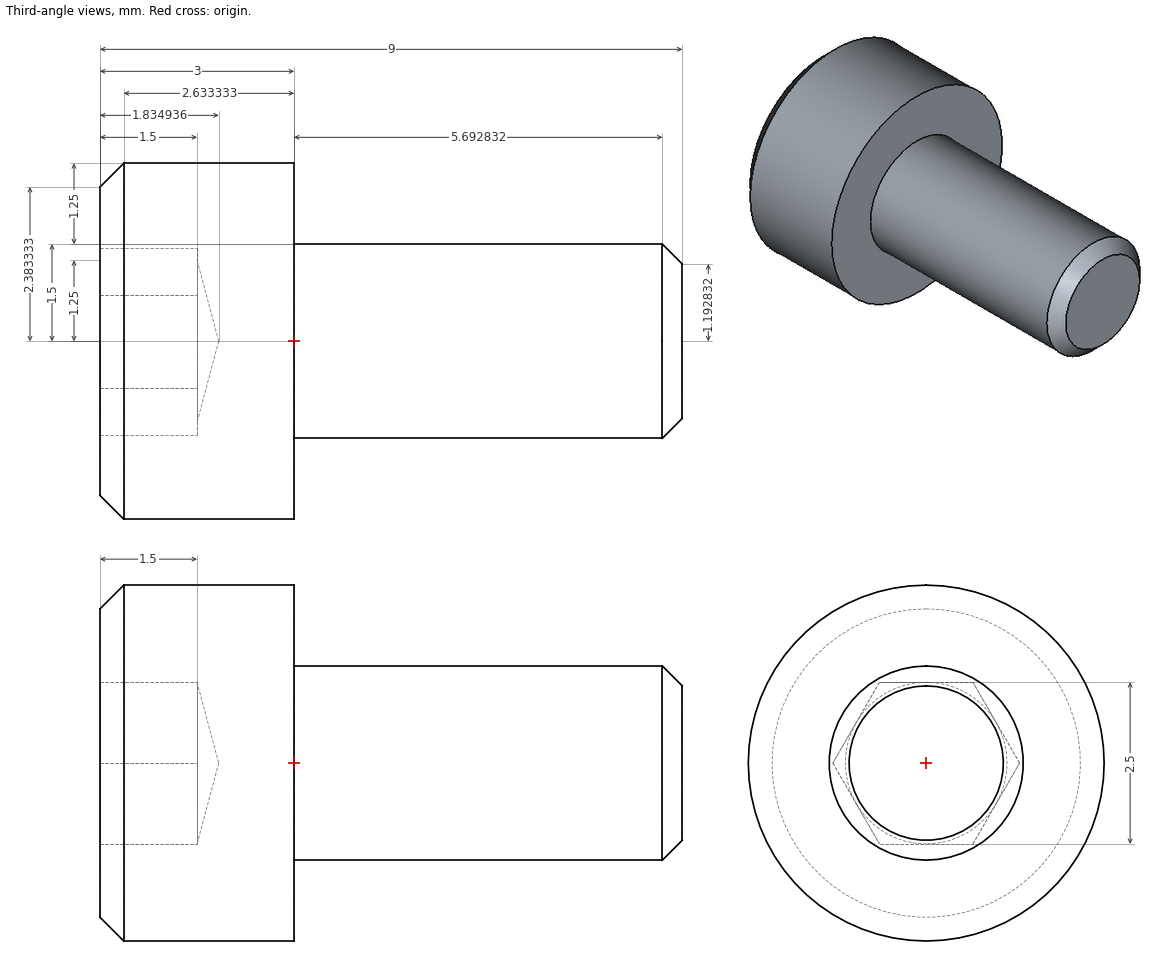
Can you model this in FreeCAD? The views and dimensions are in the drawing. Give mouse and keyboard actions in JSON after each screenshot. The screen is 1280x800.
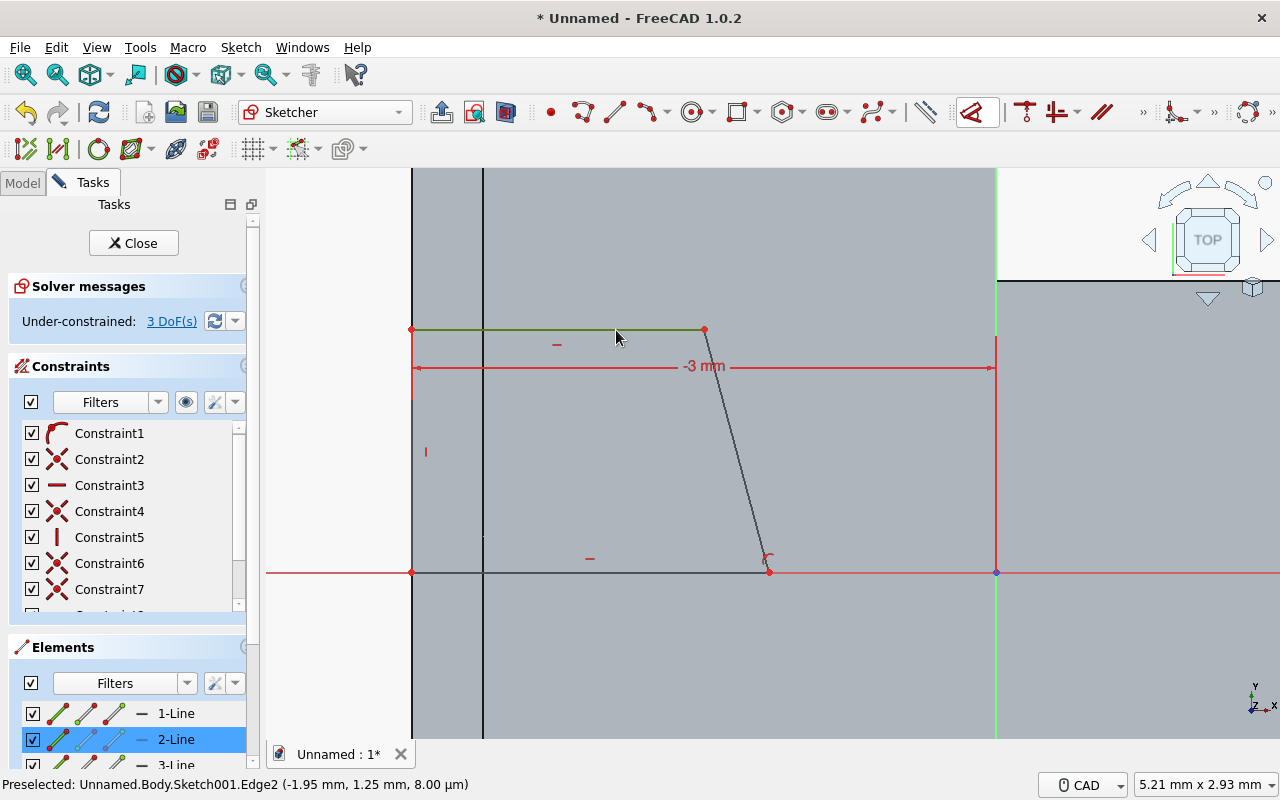
{"action": "left_click", "coordinate": [994, 112]}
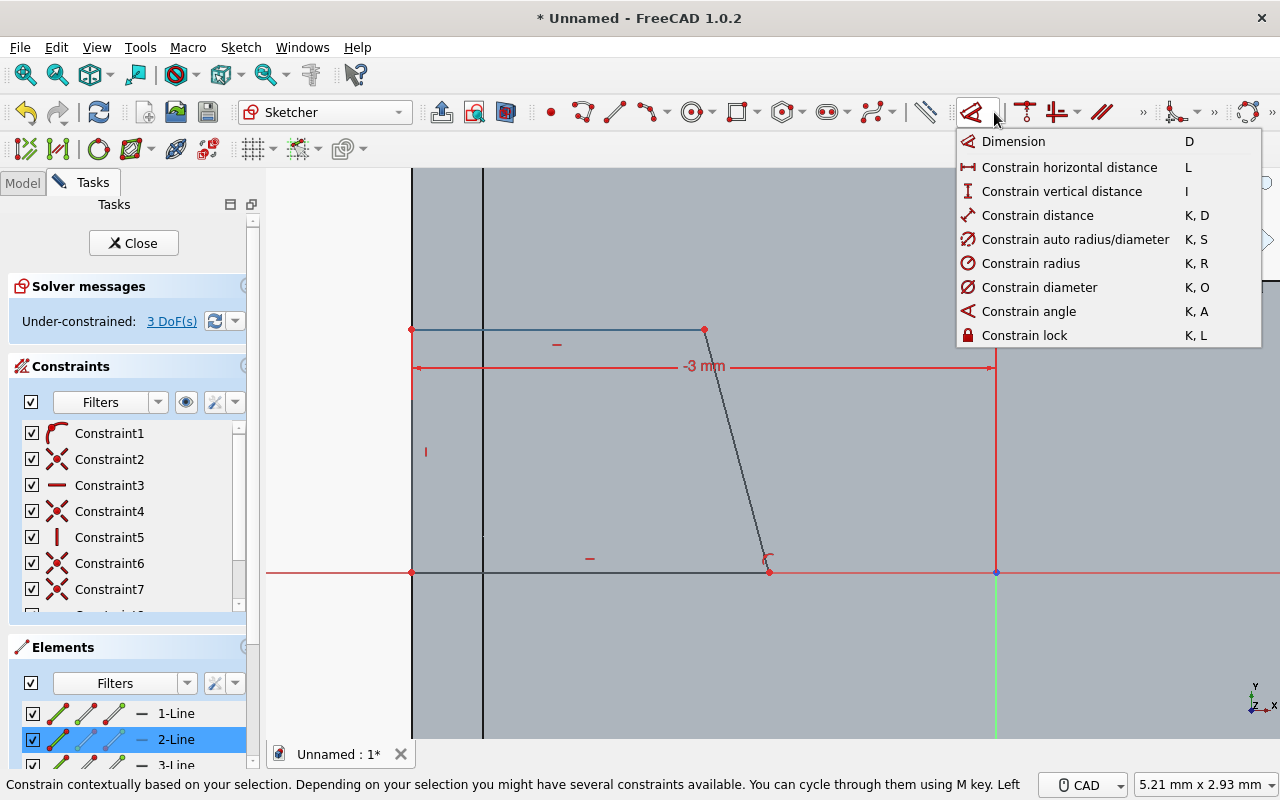
{"action": "left_click", "coordinate": [1109, 167]}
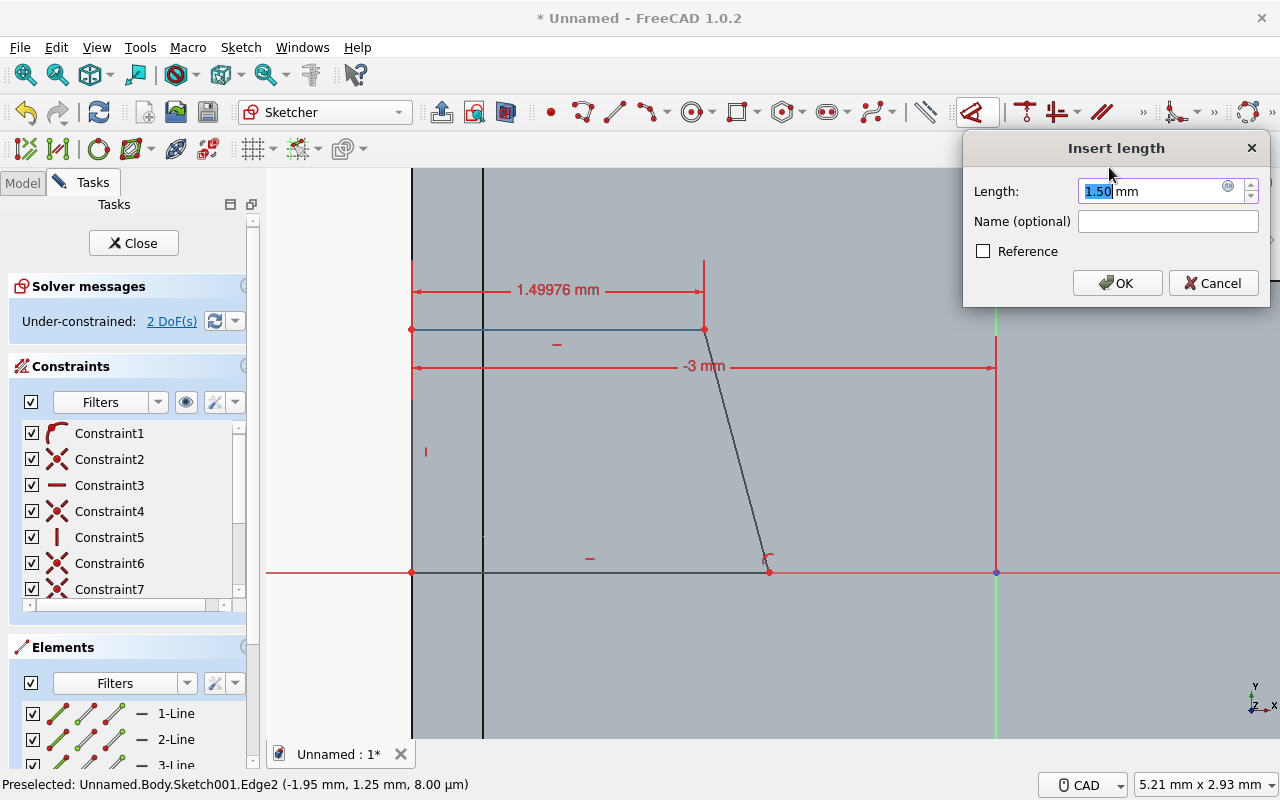
{"action": "type", "text": "1.5"}
{"action": "key", "text": "Return"}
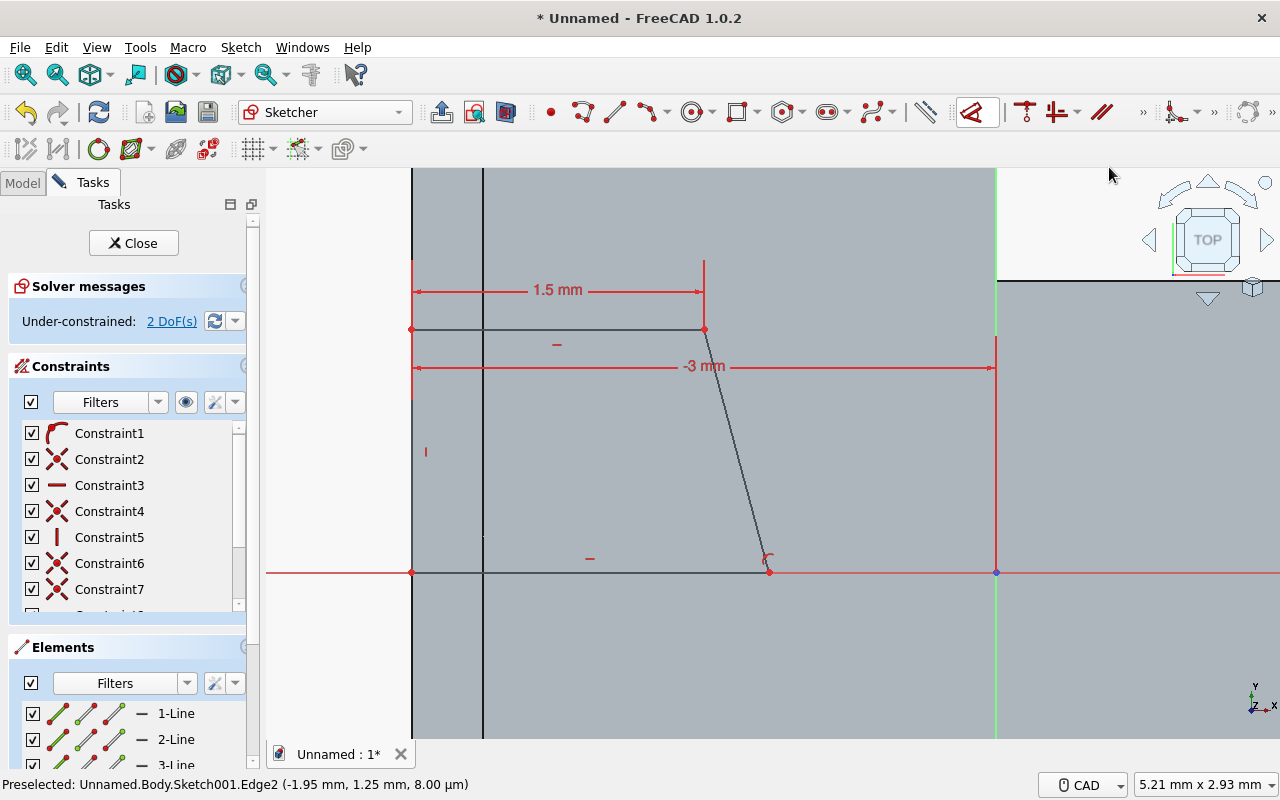
{"action": "left_click", "coordinate": [412, 403]}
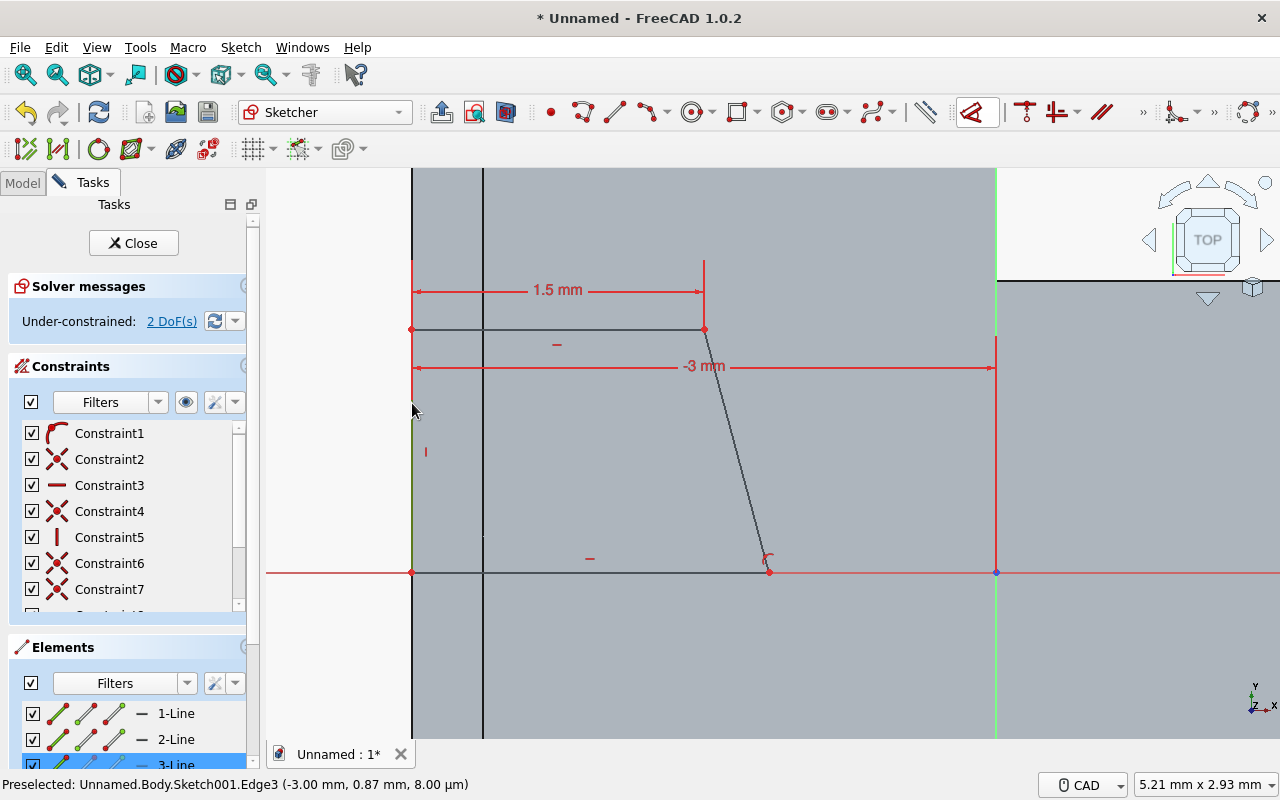
{"action": "left_click", "coordinate": [994, 112]}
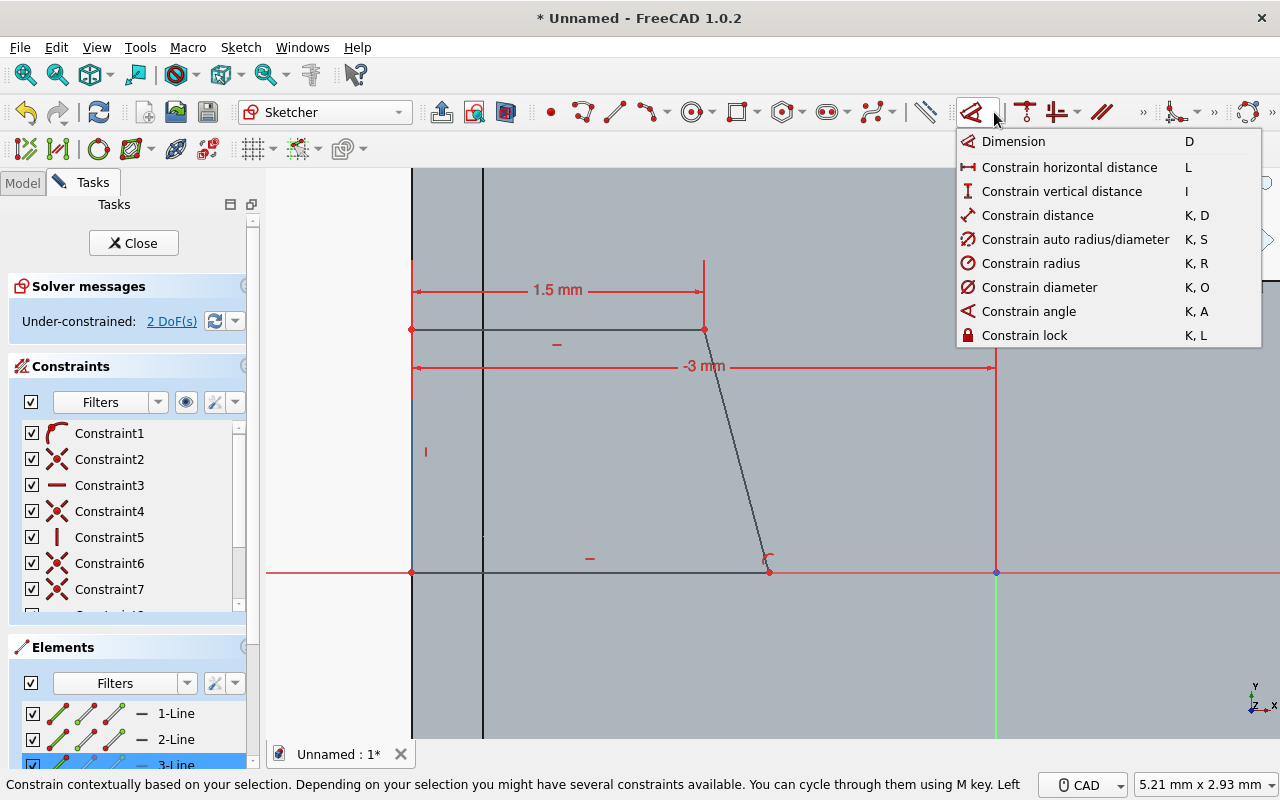
{"action": "left_click", "coordinate": [1109, 191]}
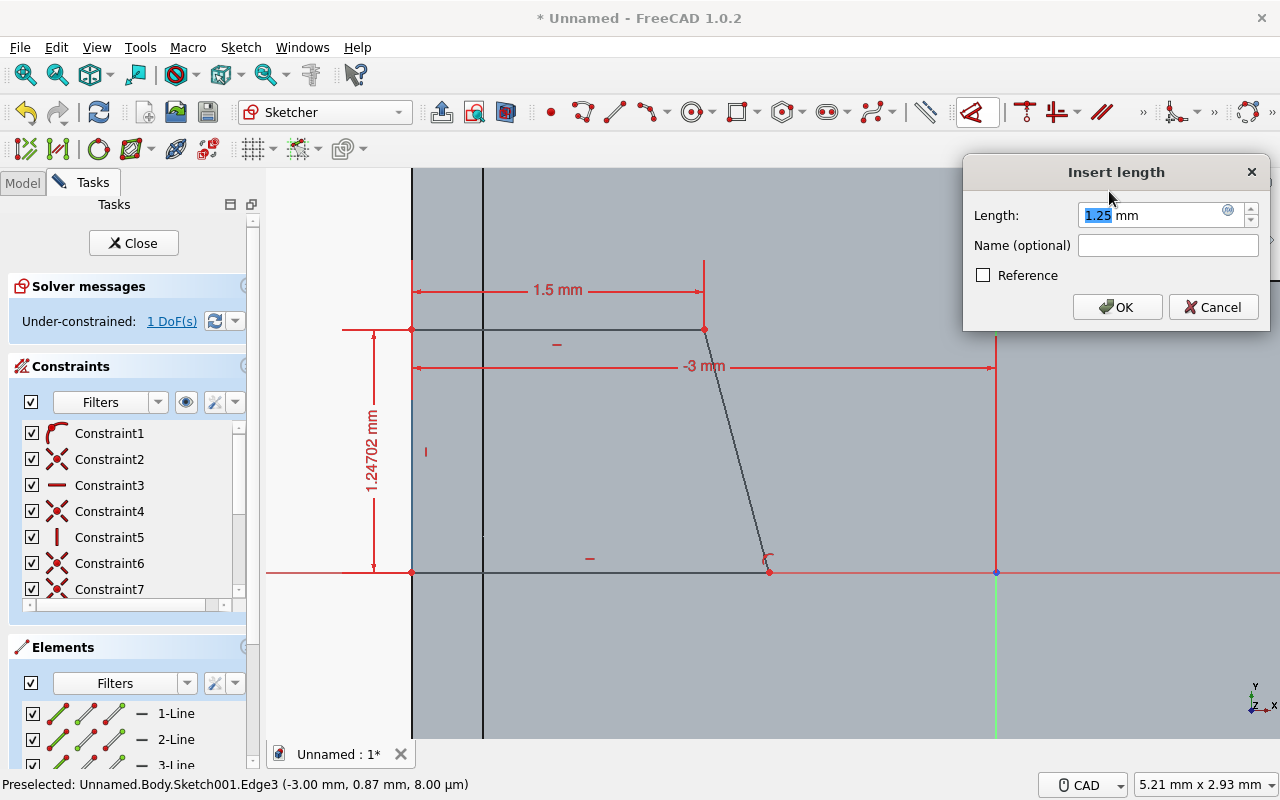
{"action": "type", "text": "1.25"}
{"action": "key", "text": "Return"}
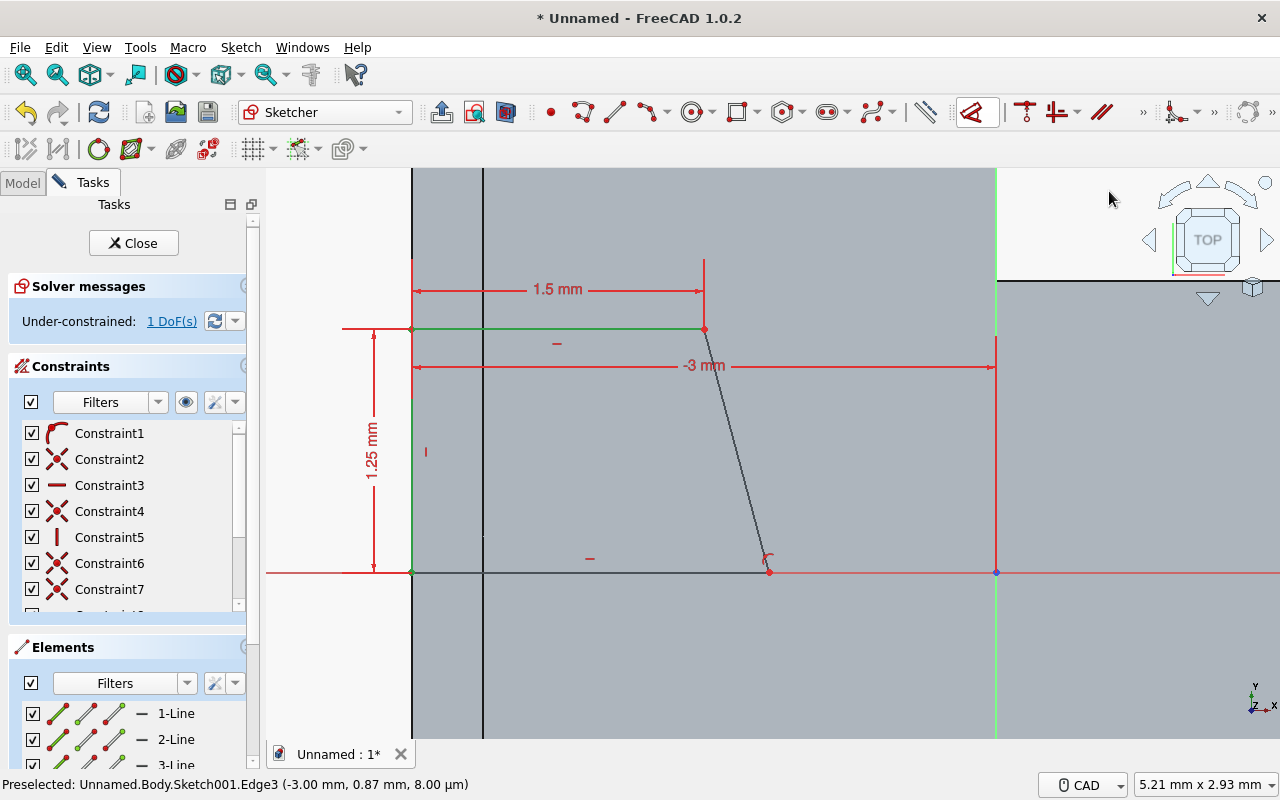
{"action": "left_click", "coordinate": [519, 573]}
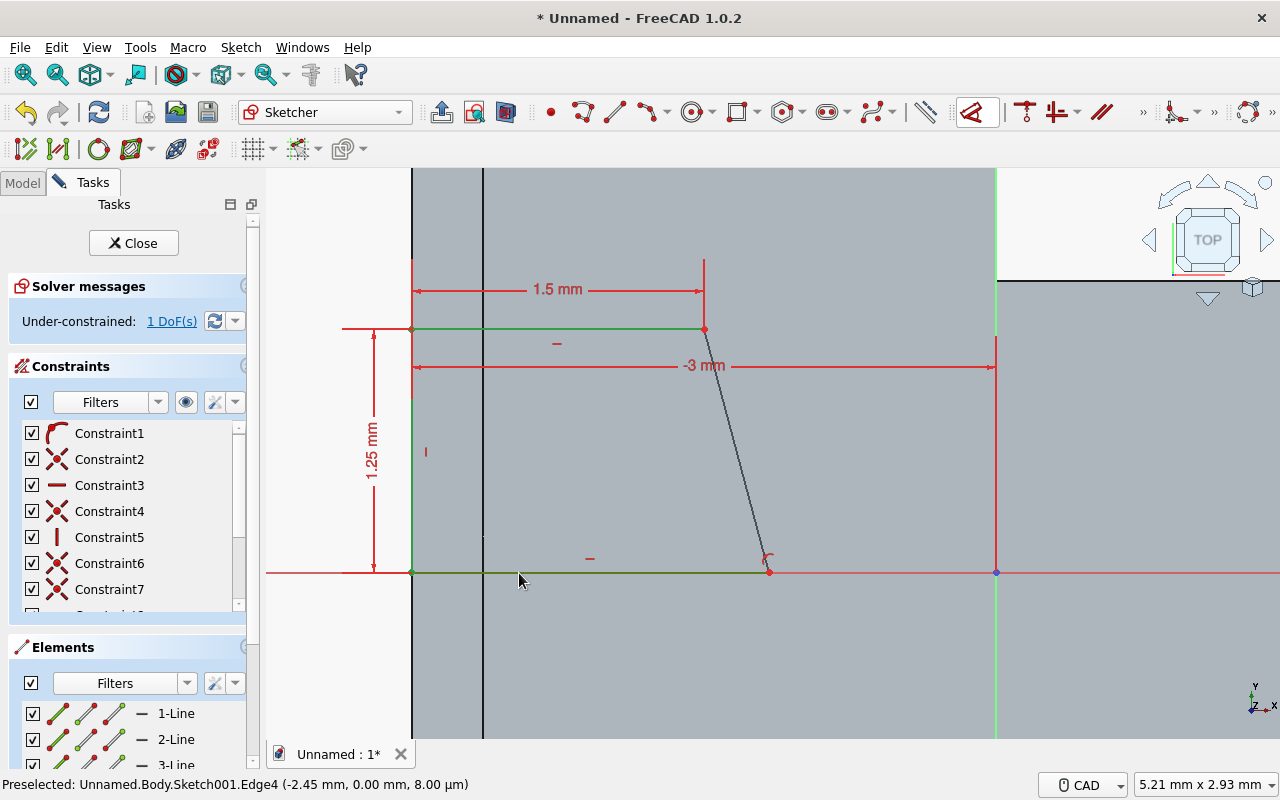
{"action": "left_click", "coordinate": [994, 112]}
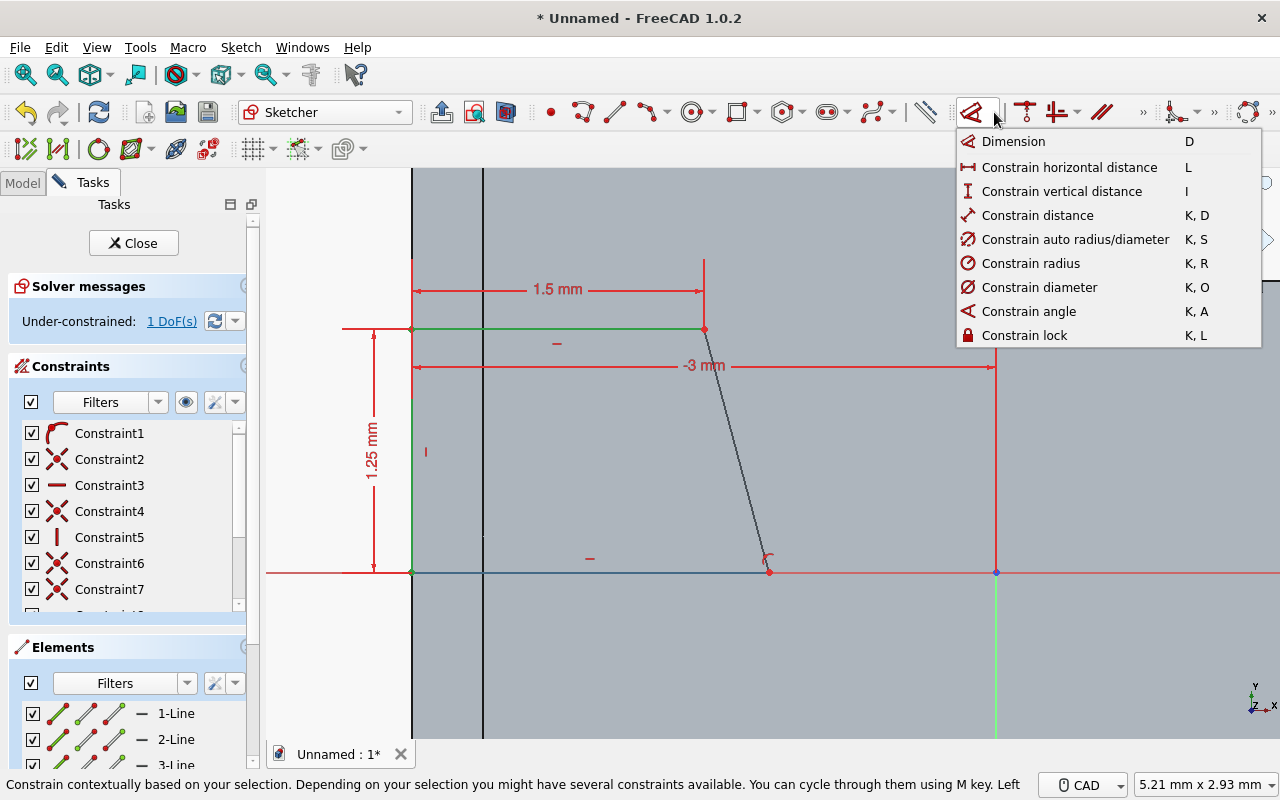
{"action": "left_click", "coordinate": [1109, 167]}